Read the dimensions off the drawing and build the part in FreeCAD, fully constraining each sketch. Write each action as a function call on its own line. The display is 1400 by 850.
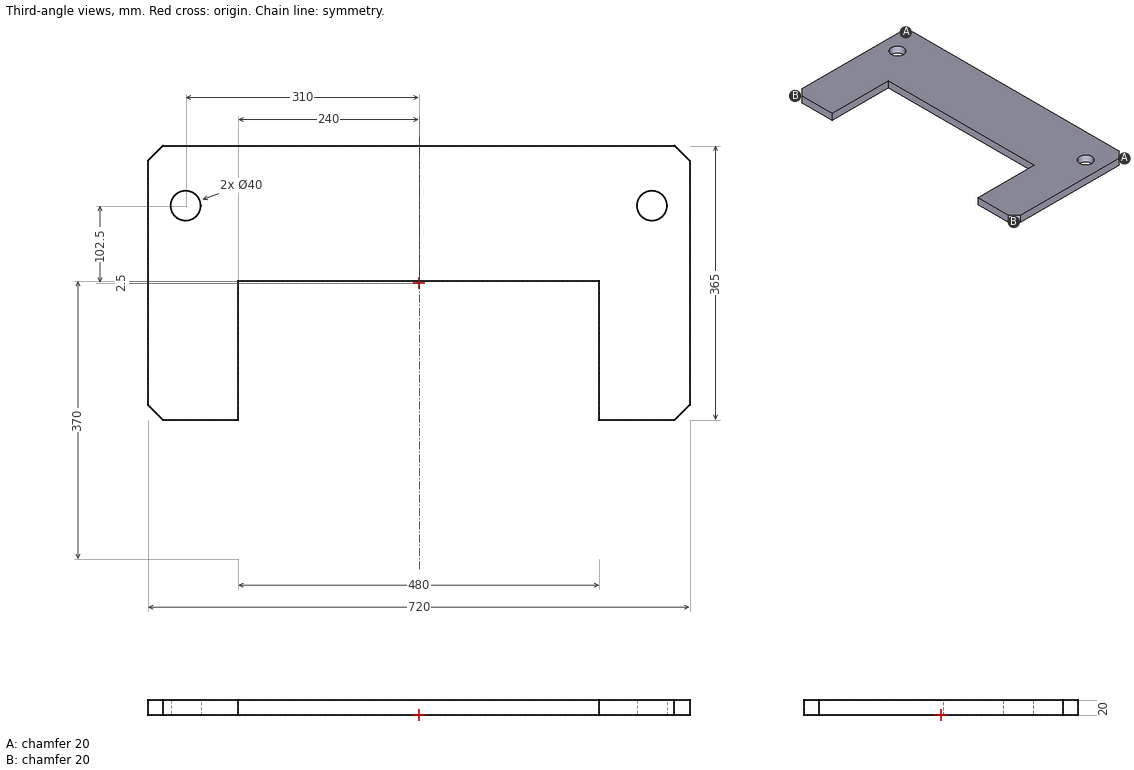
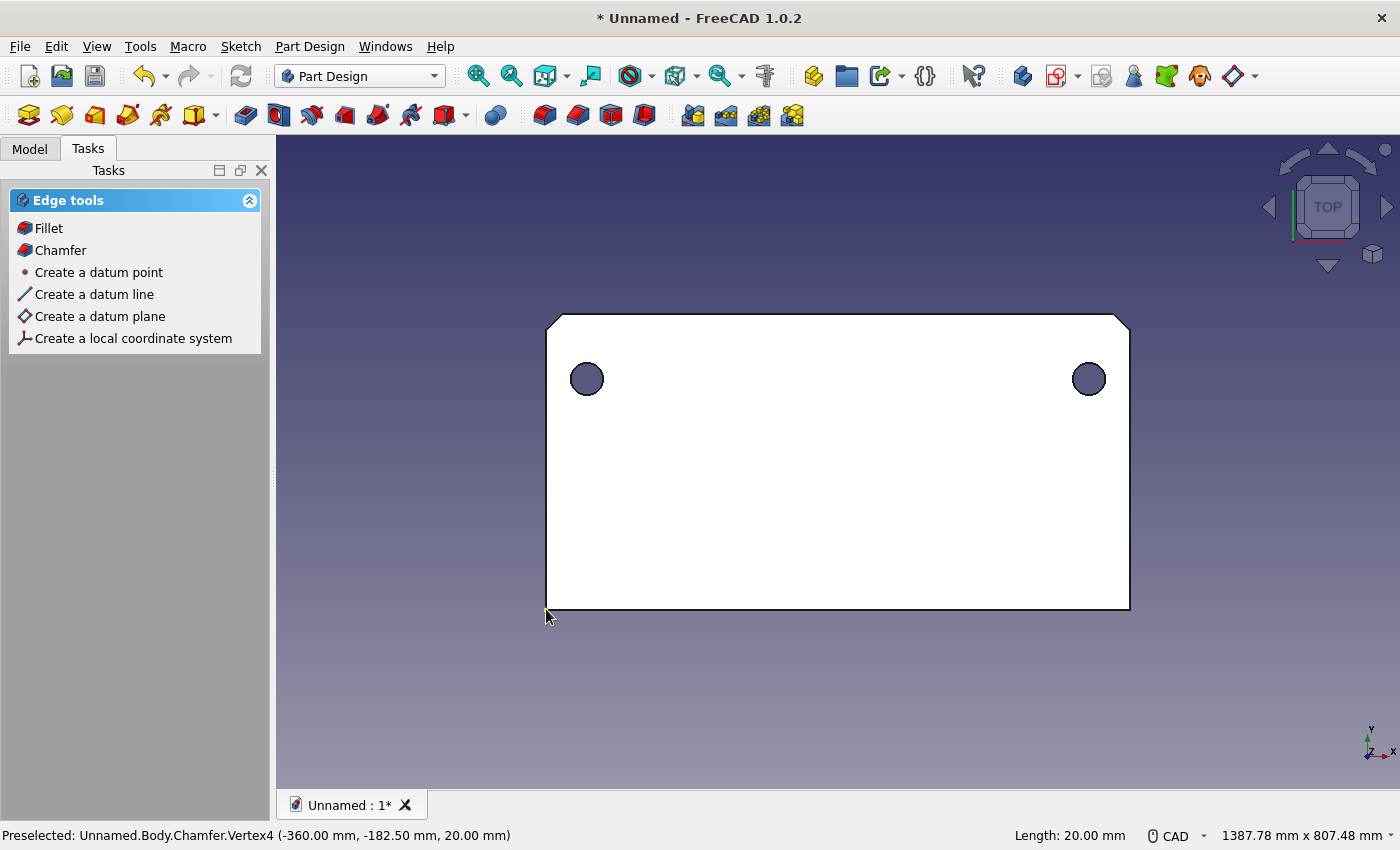
key(1)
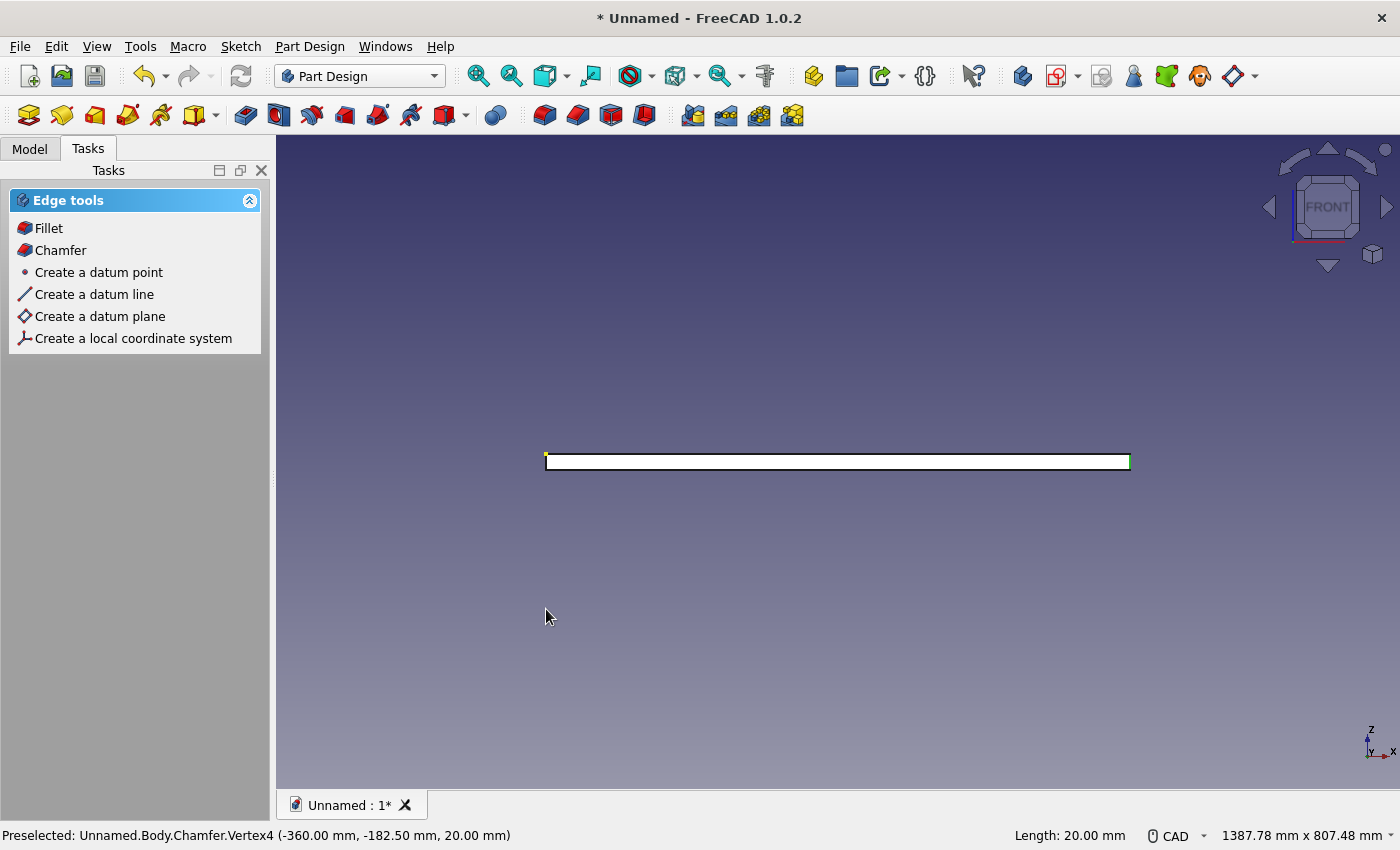
click(546, 461, ctrl)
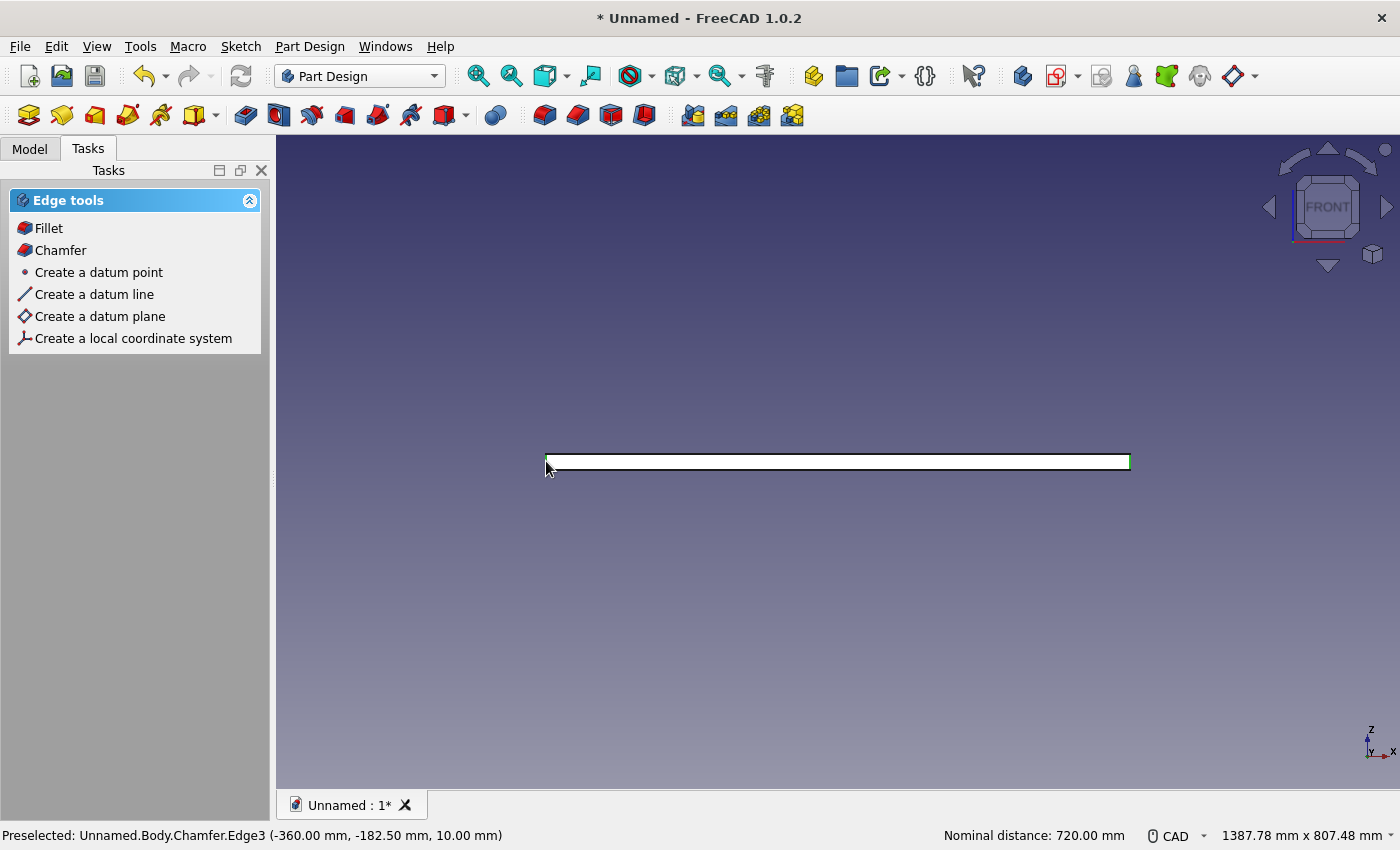
click(578, 116)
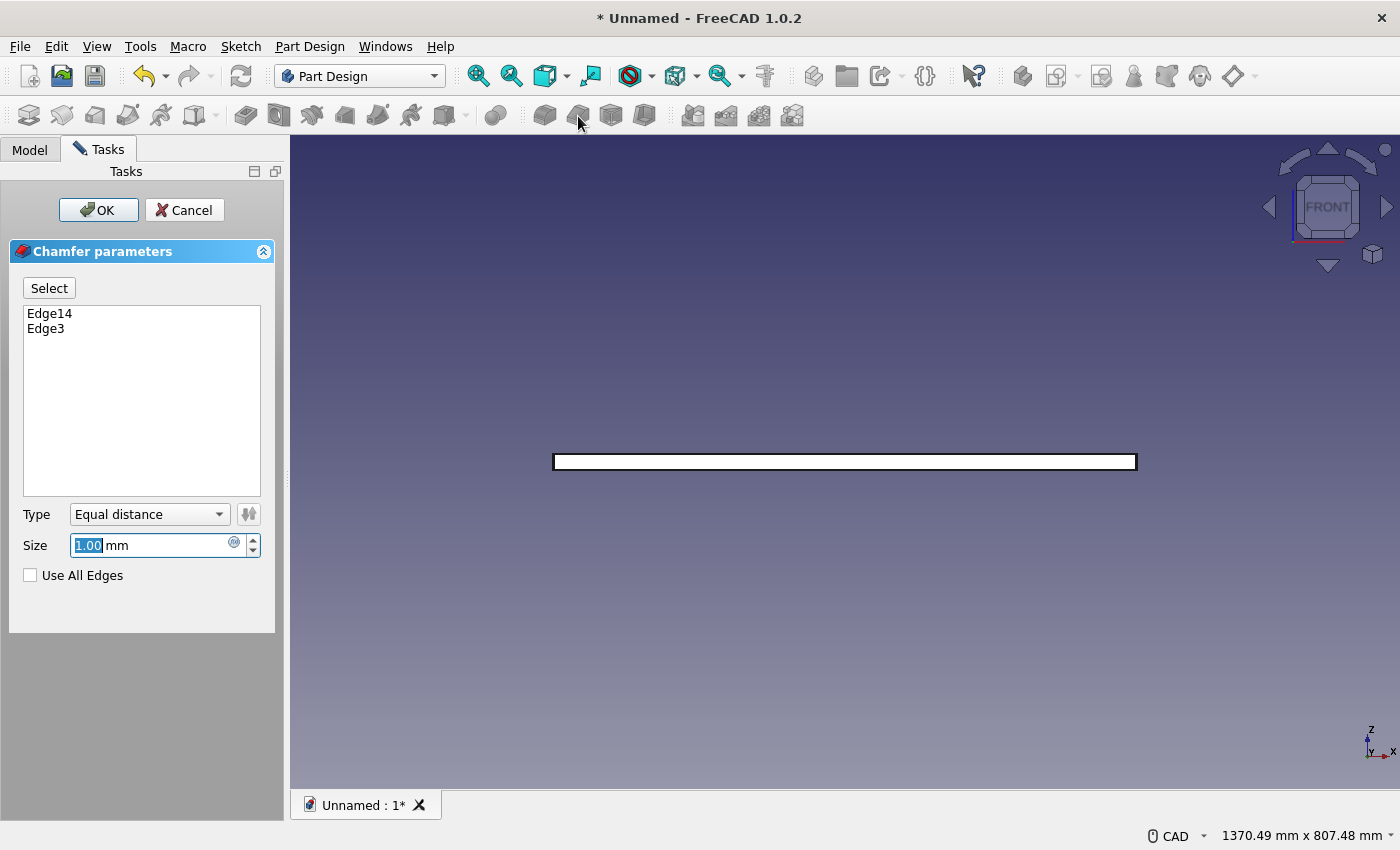
text(20)
key(Tab)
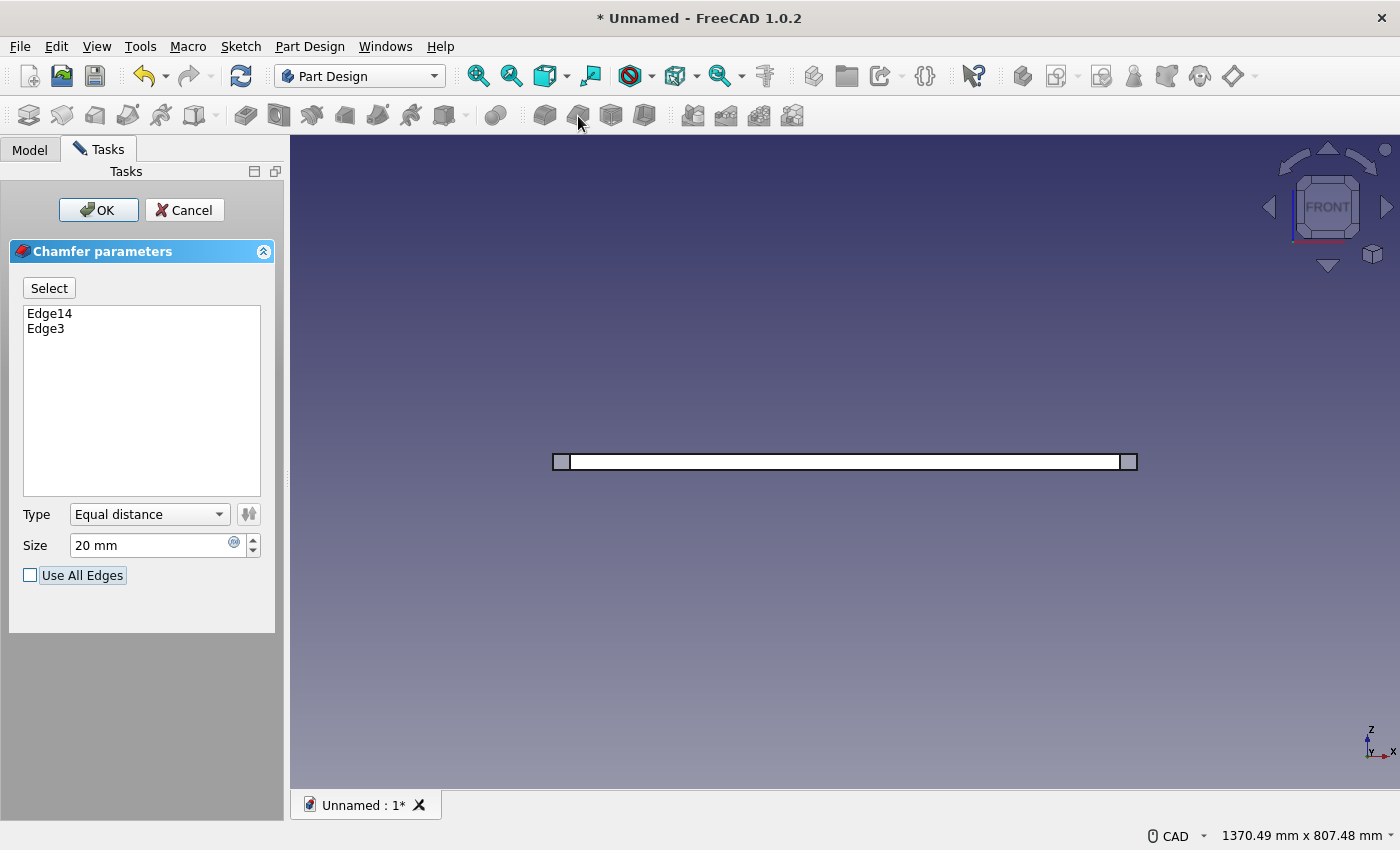
click(99, 210)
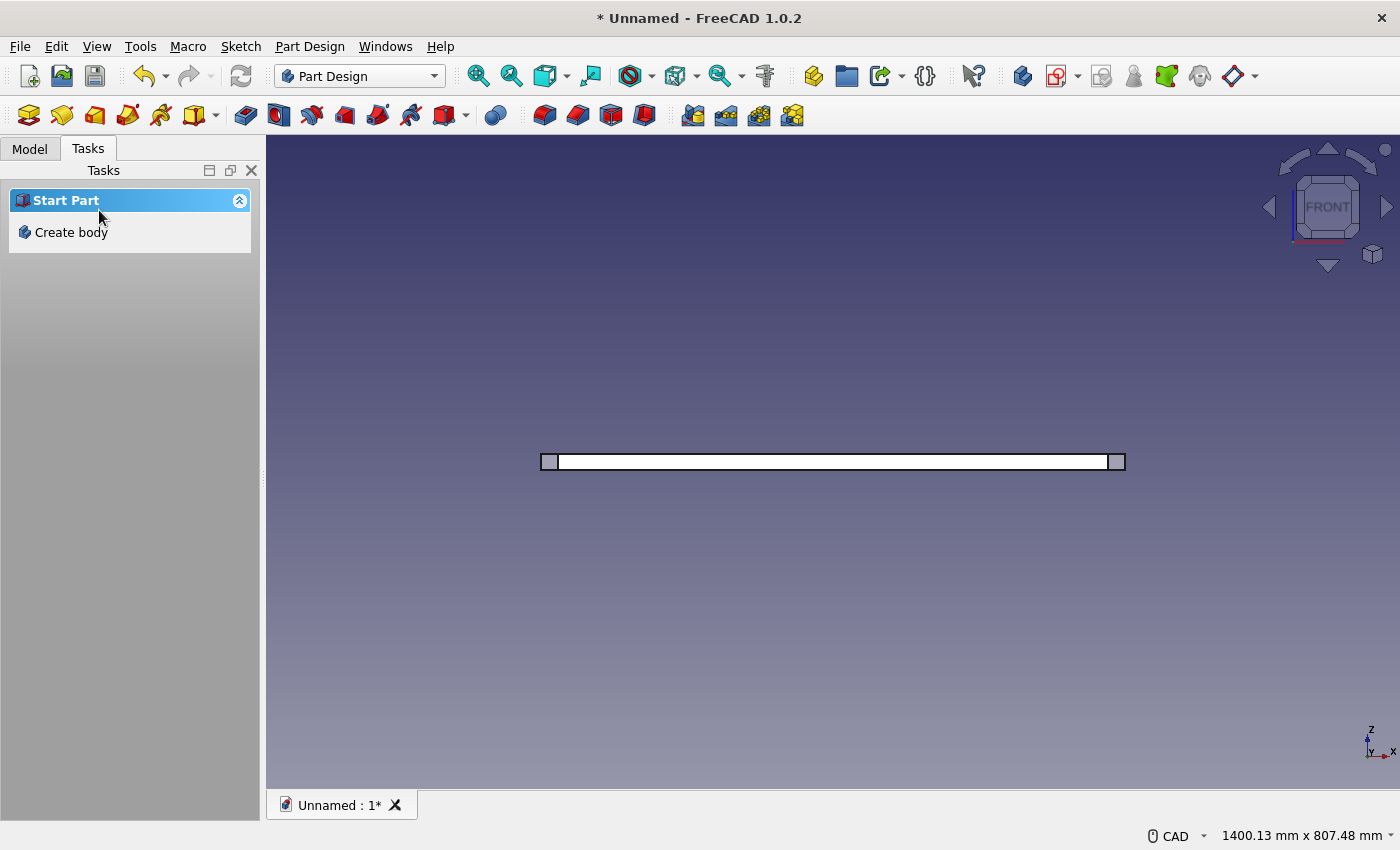
key(0)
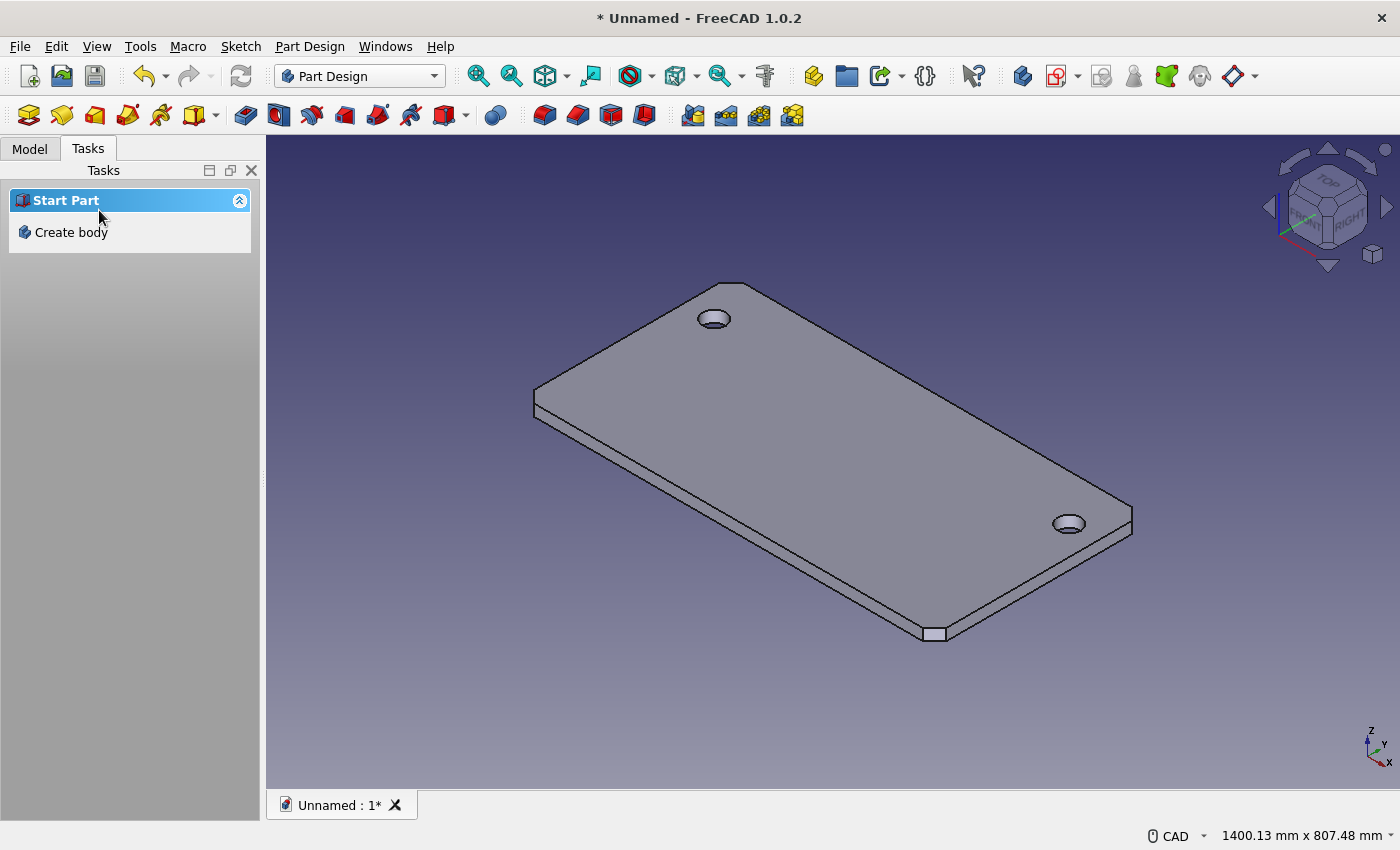
click(892, 488)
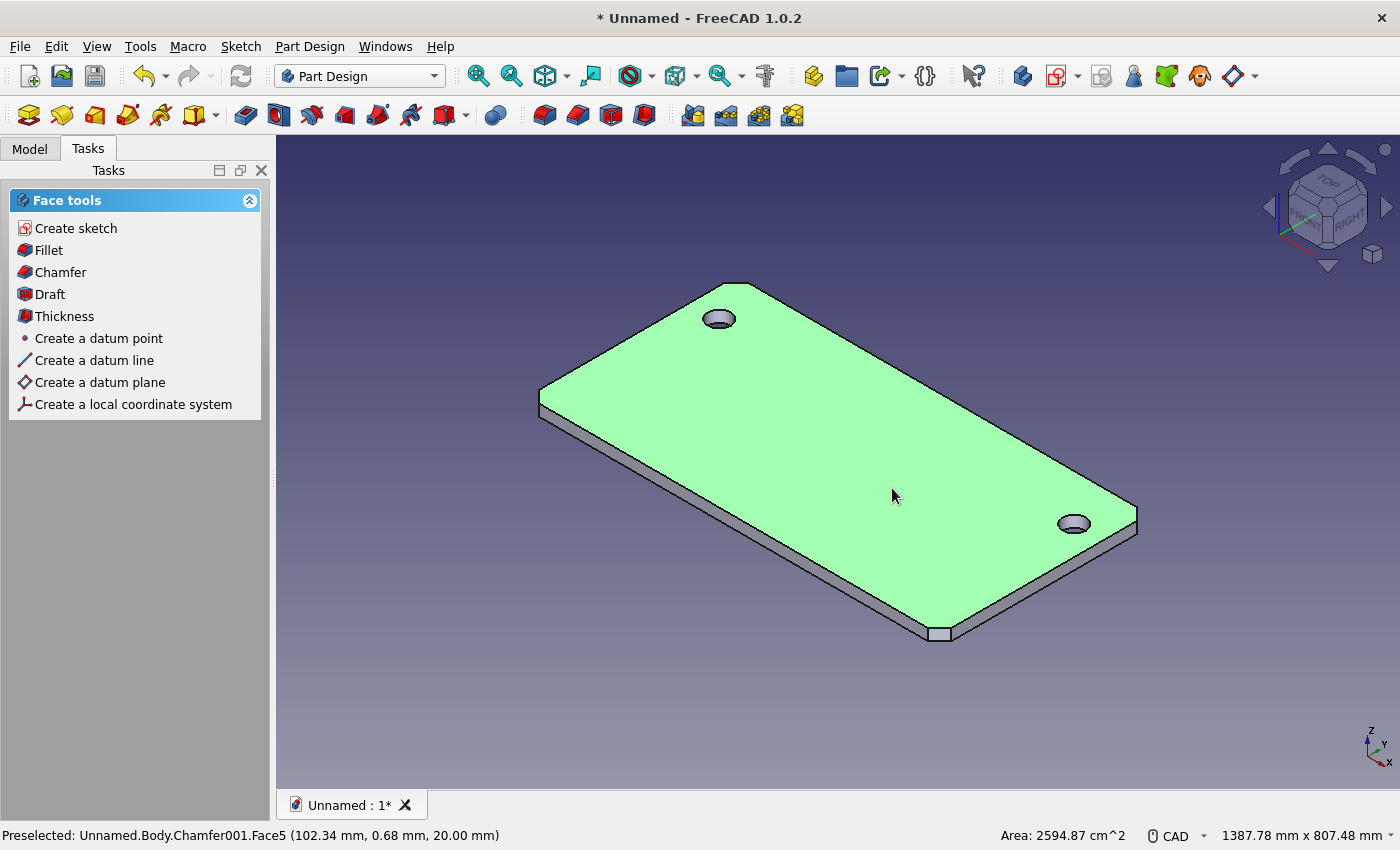
click(1056, 76)